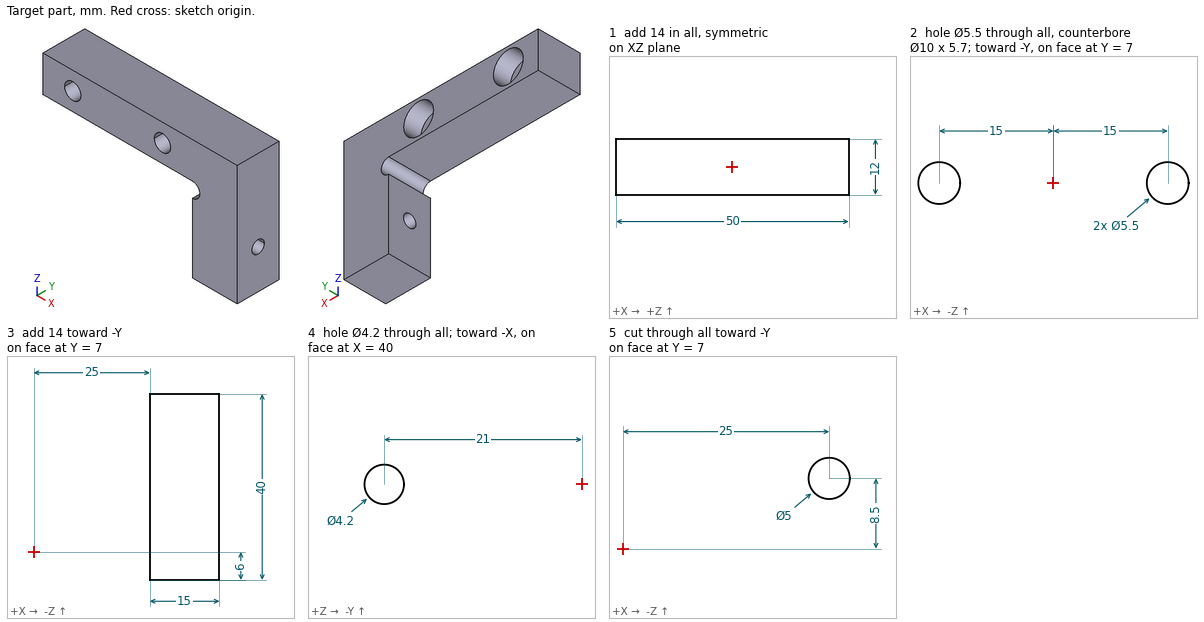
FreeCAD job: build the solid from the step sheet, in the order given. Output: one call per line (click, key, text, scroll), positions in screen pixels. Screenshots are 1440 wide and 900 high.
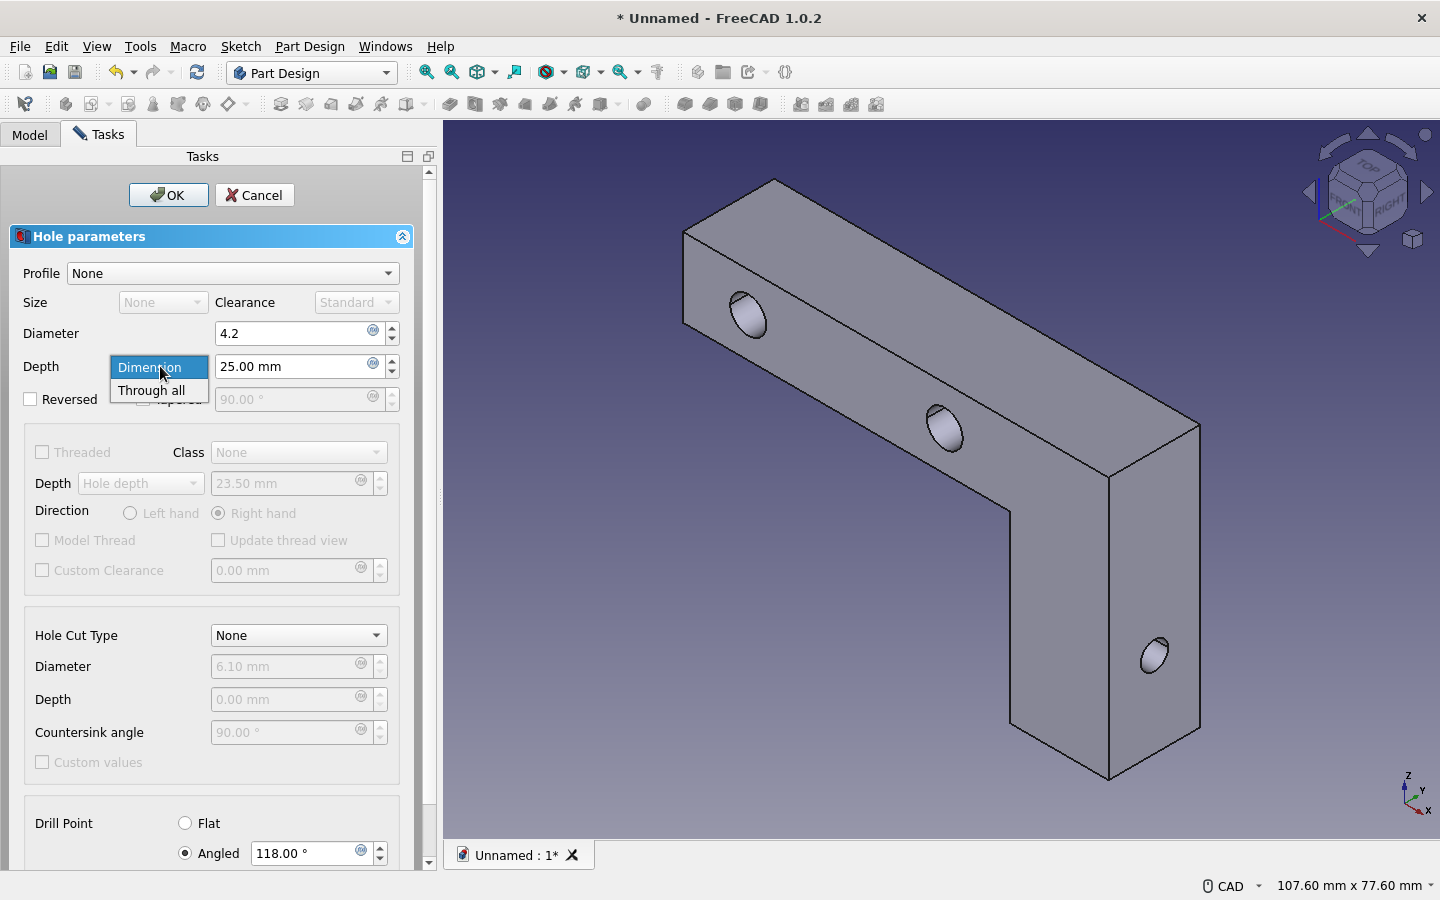
click(158, 390)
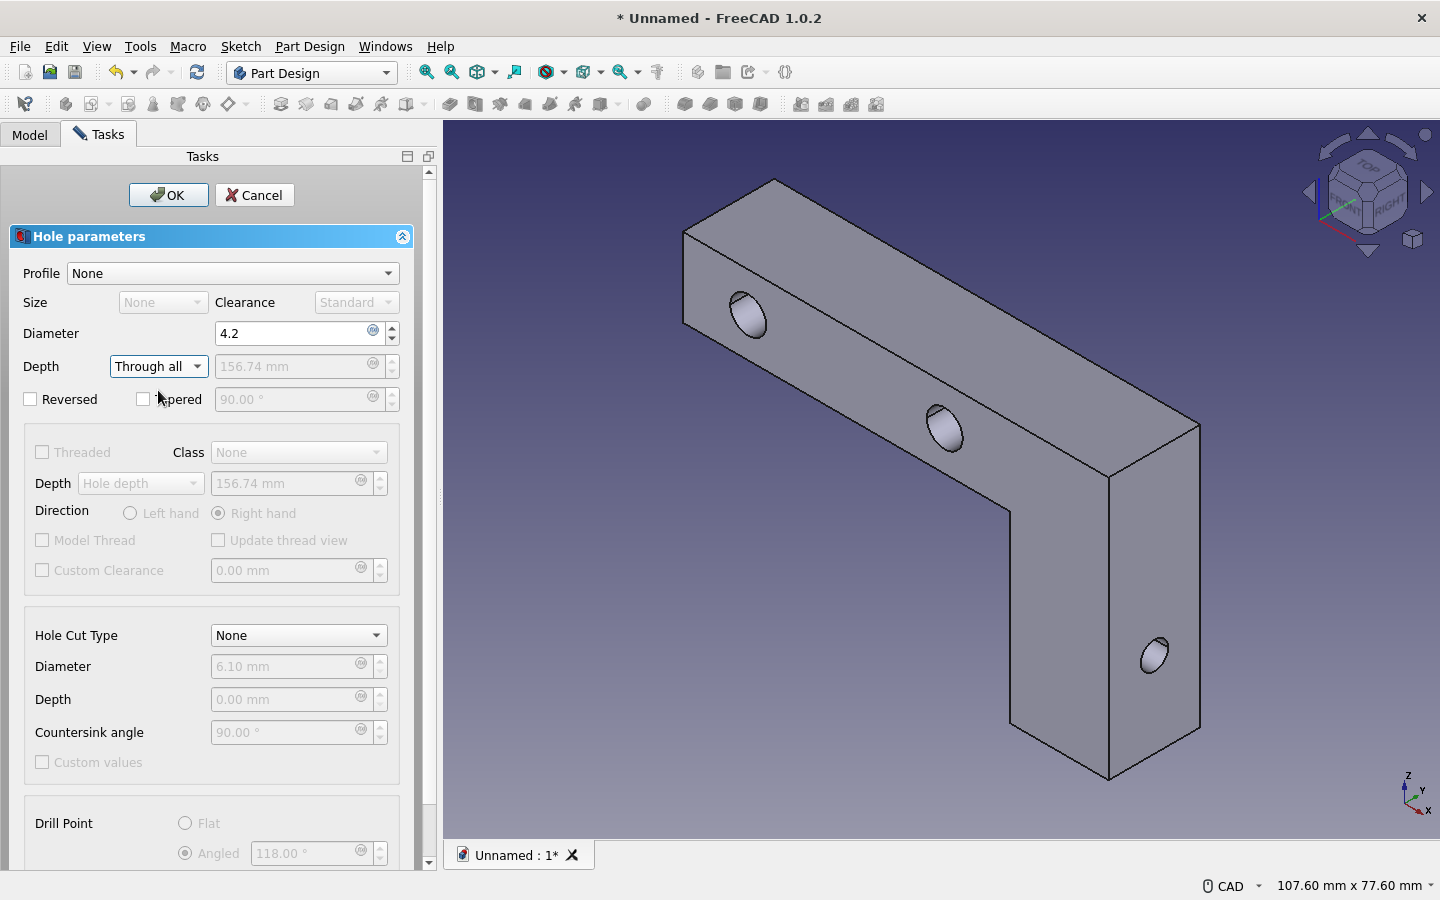
click(169, 195)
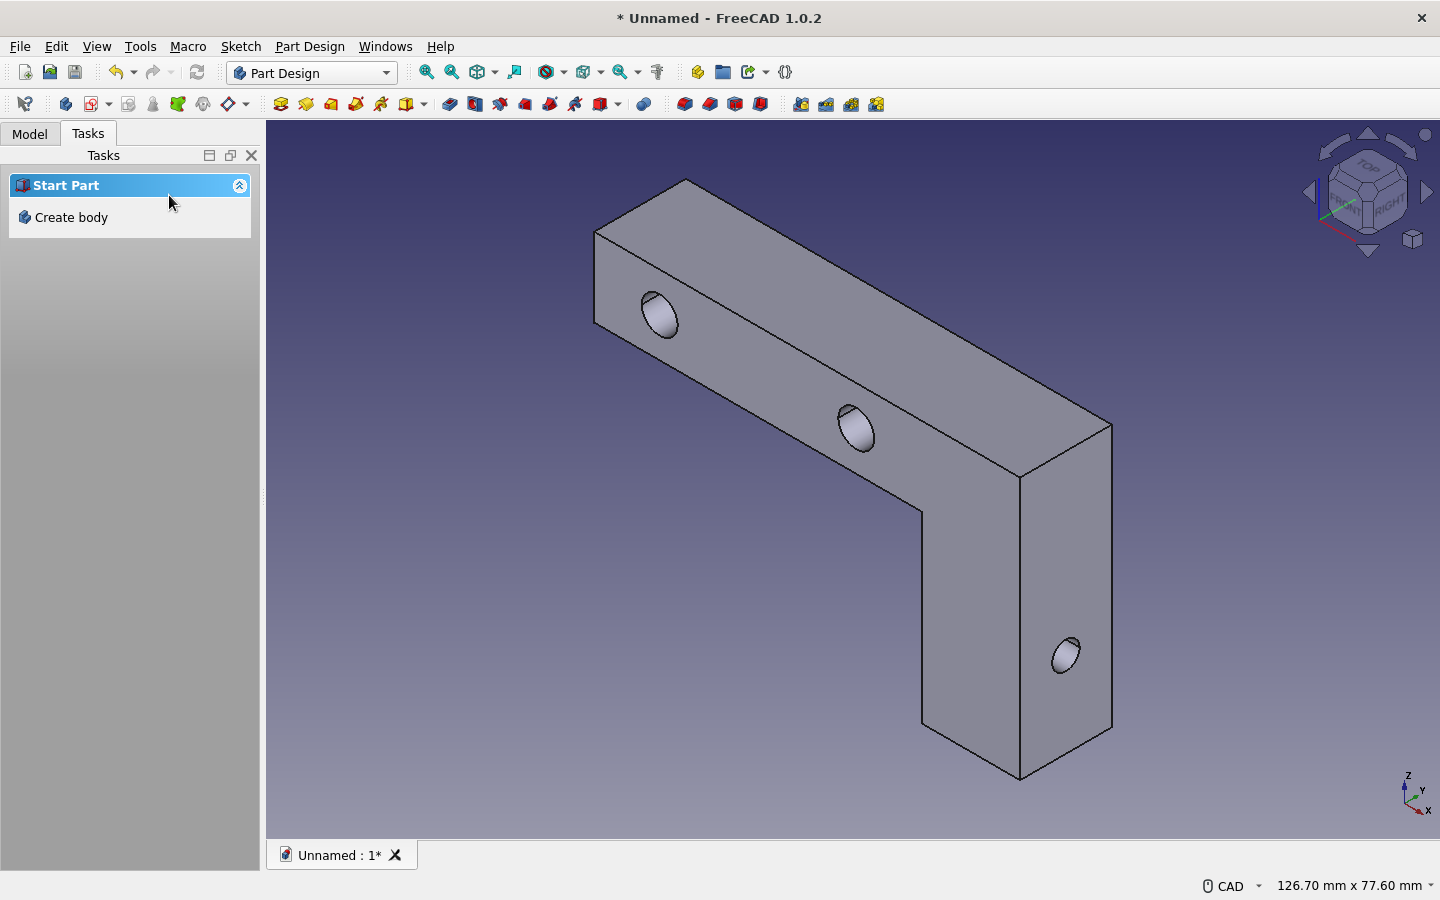
key(4)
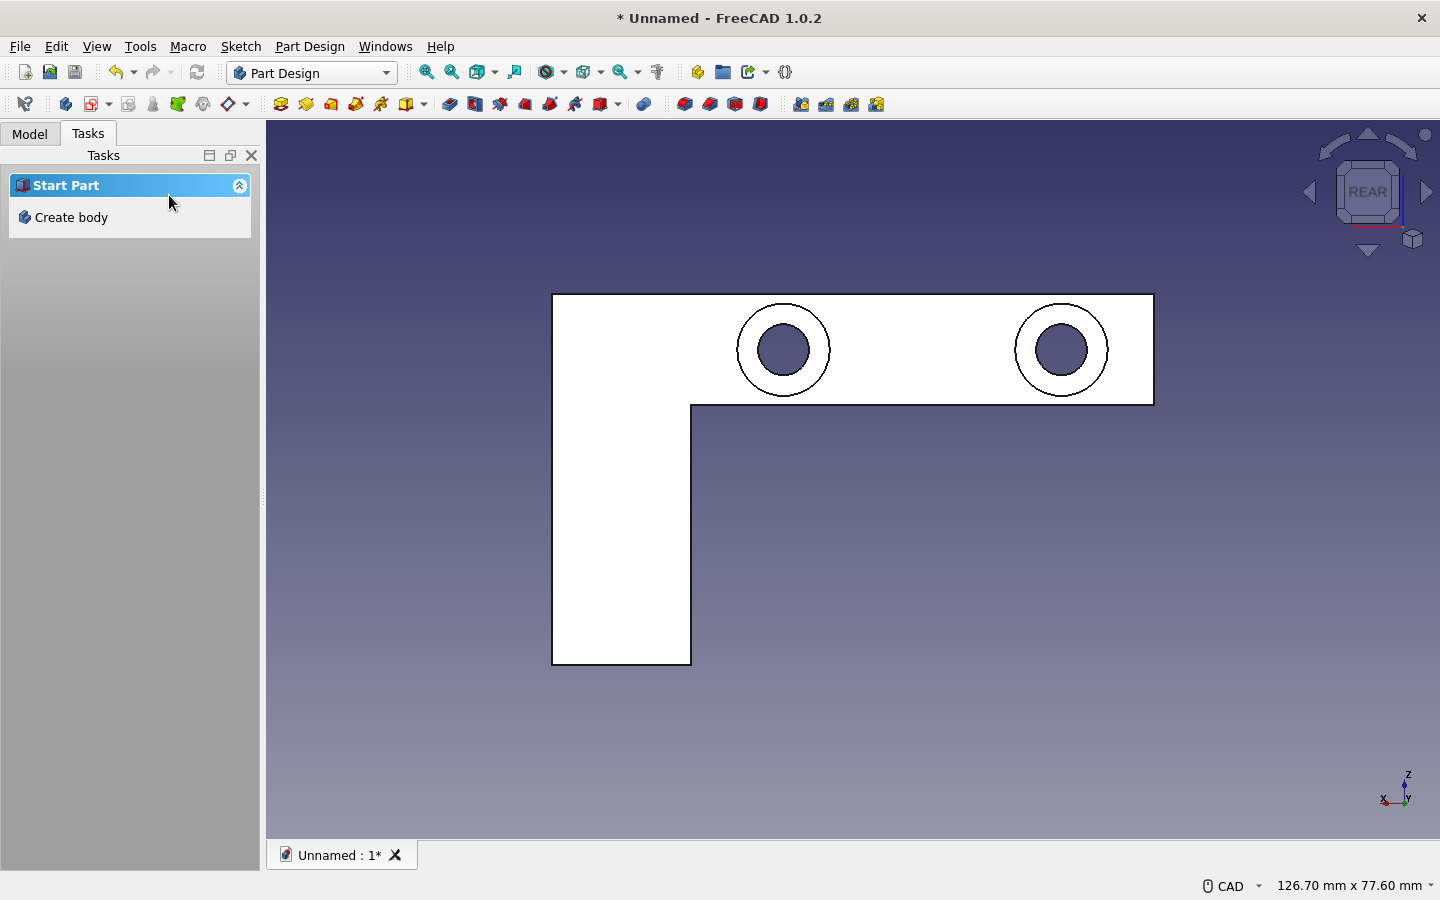
click(595, 584)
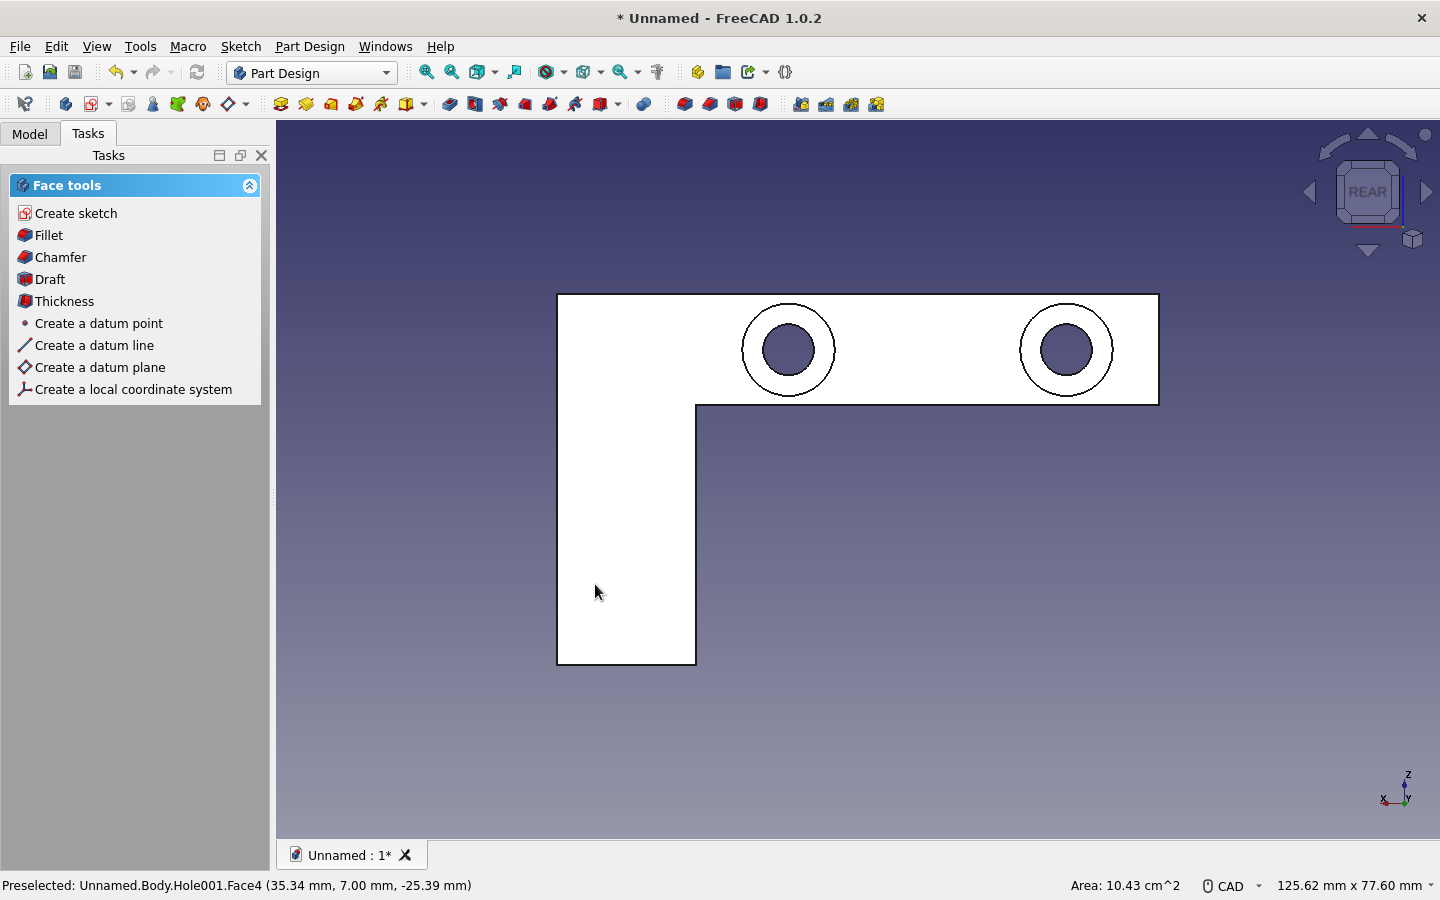
click(90, 104)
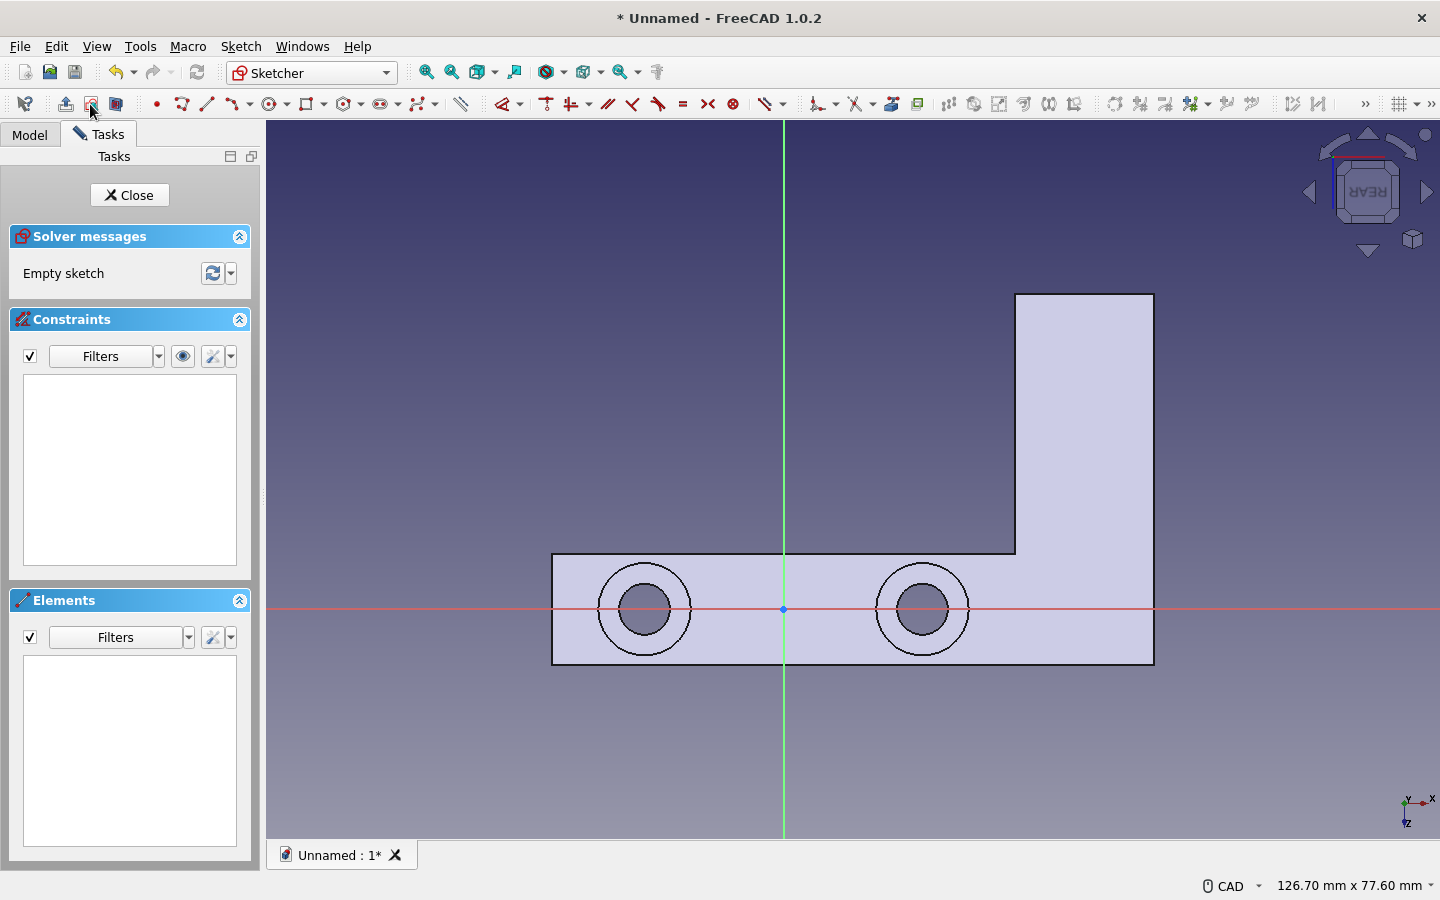
scroll(1038, 536, up, 12)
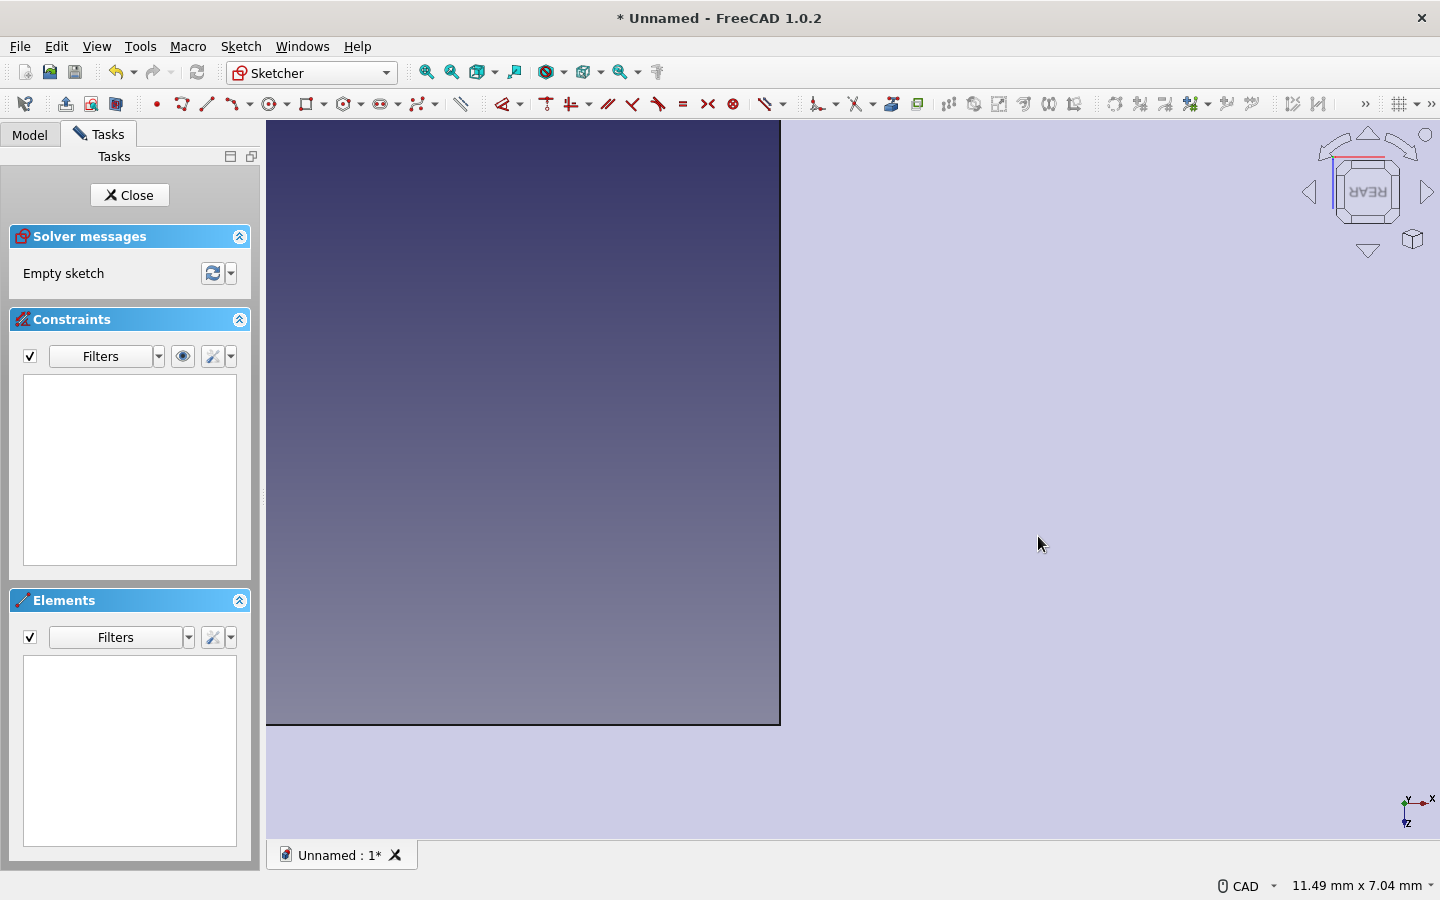
click(268, 104)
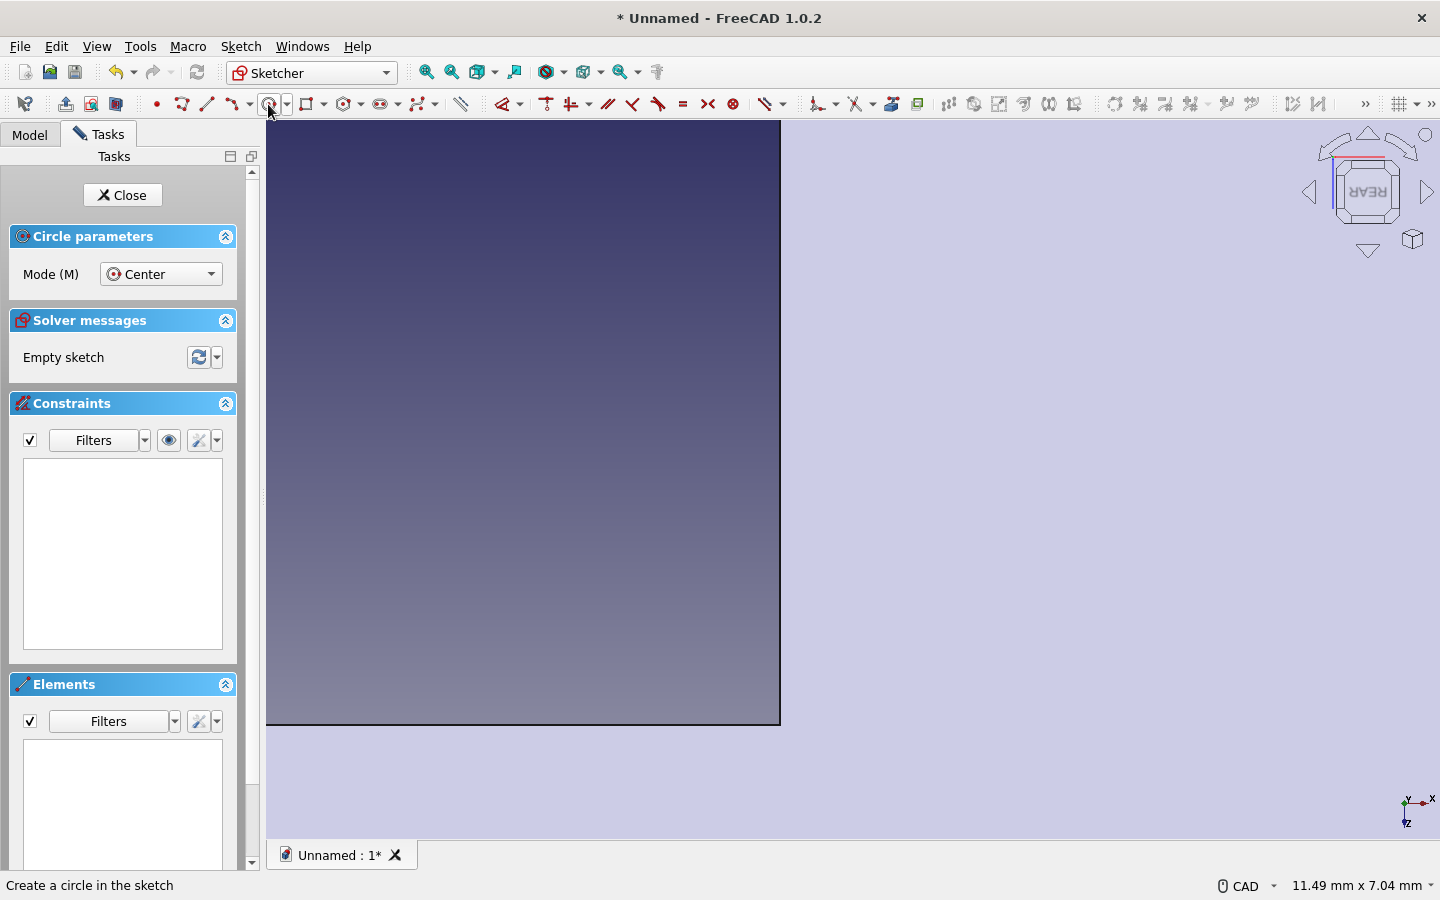
click(780, 469)
move(960, 289)